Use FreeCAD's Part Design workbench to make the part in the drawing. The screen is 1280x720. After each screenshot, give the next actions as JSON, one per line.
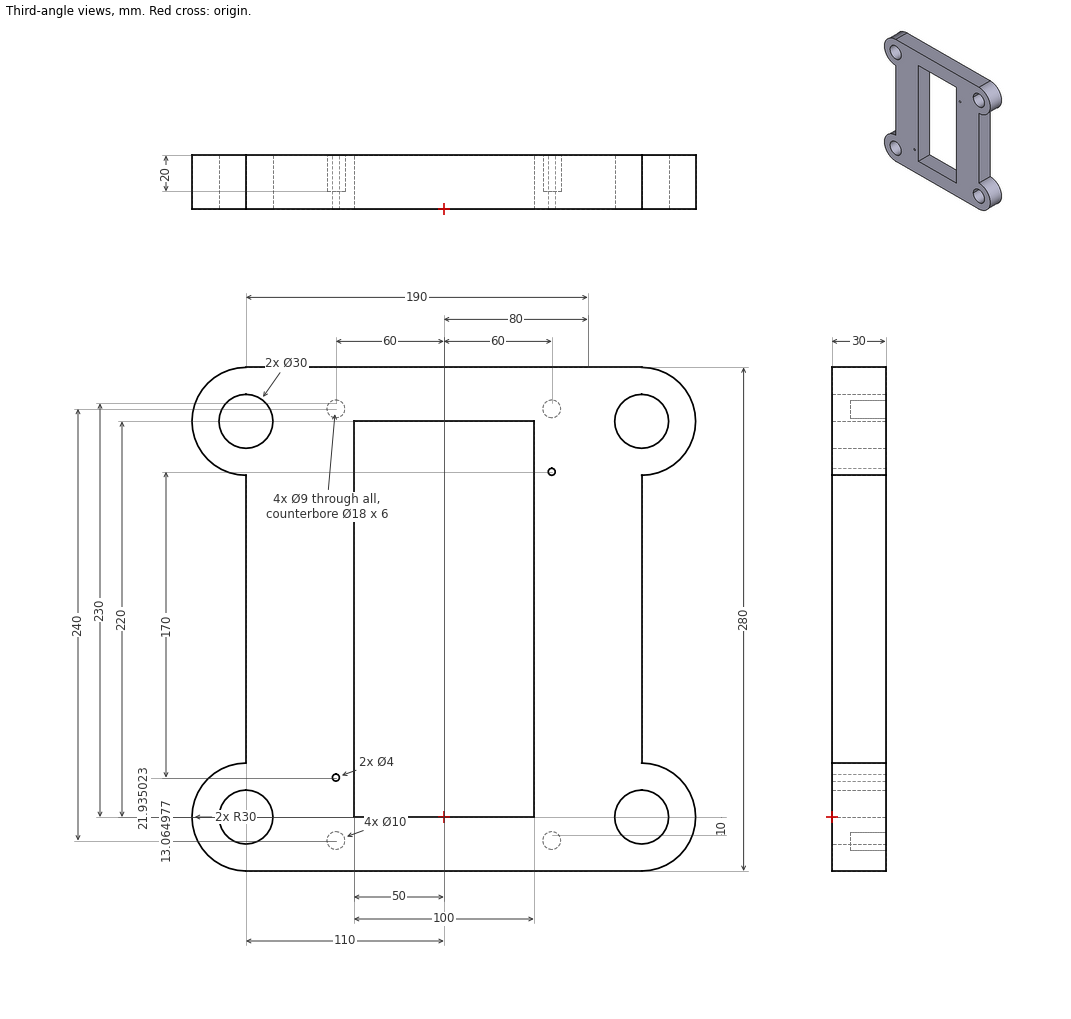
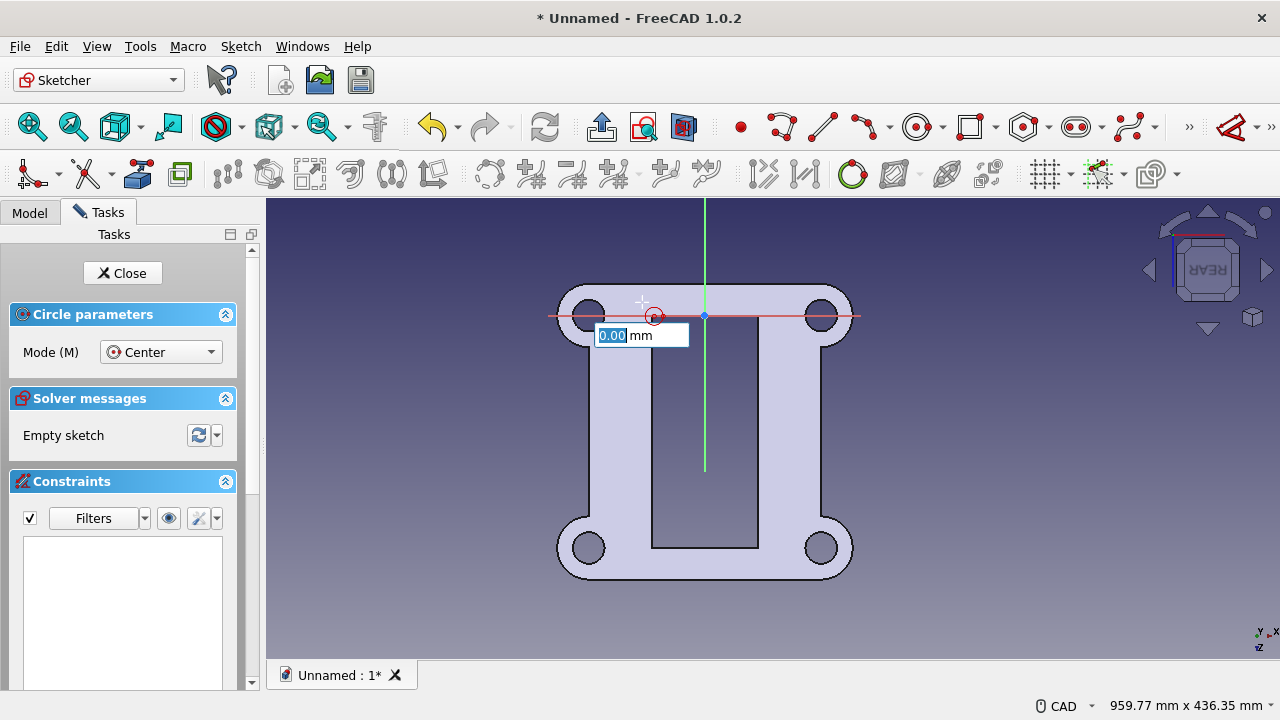
{"action": "scroll", "coordinate": [645, 298], "scroll_direction": "up", "scroll_amount": 6}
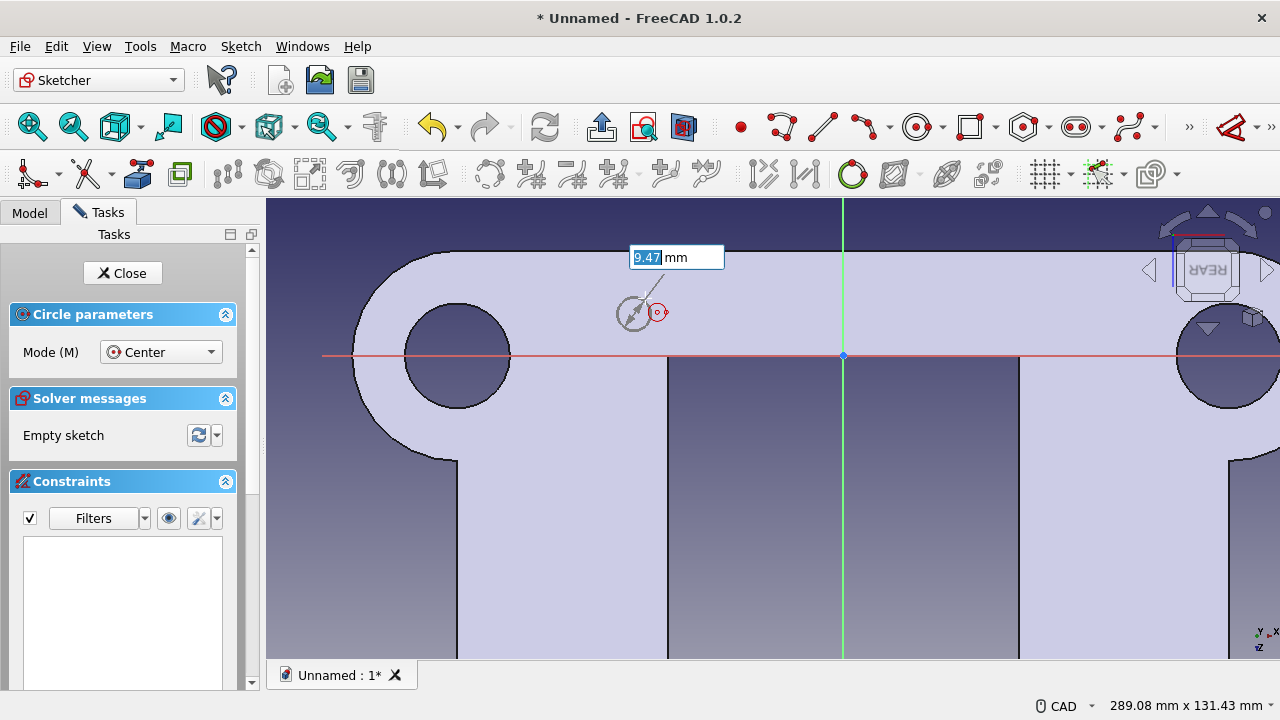
{"action": "left_click", "coordinate": [645, 298]}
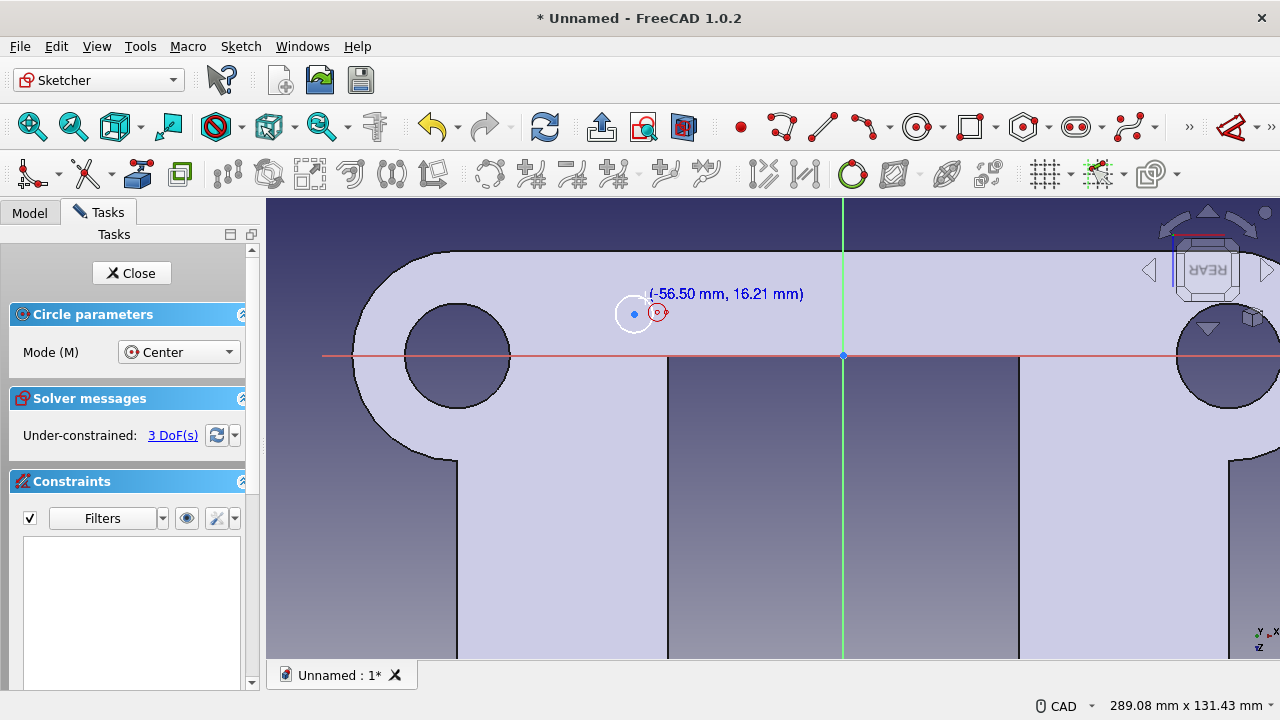
{"action": "scroll", "coordinate": [645, 298], "scroll_direction": "down", "scroll_amount": 6}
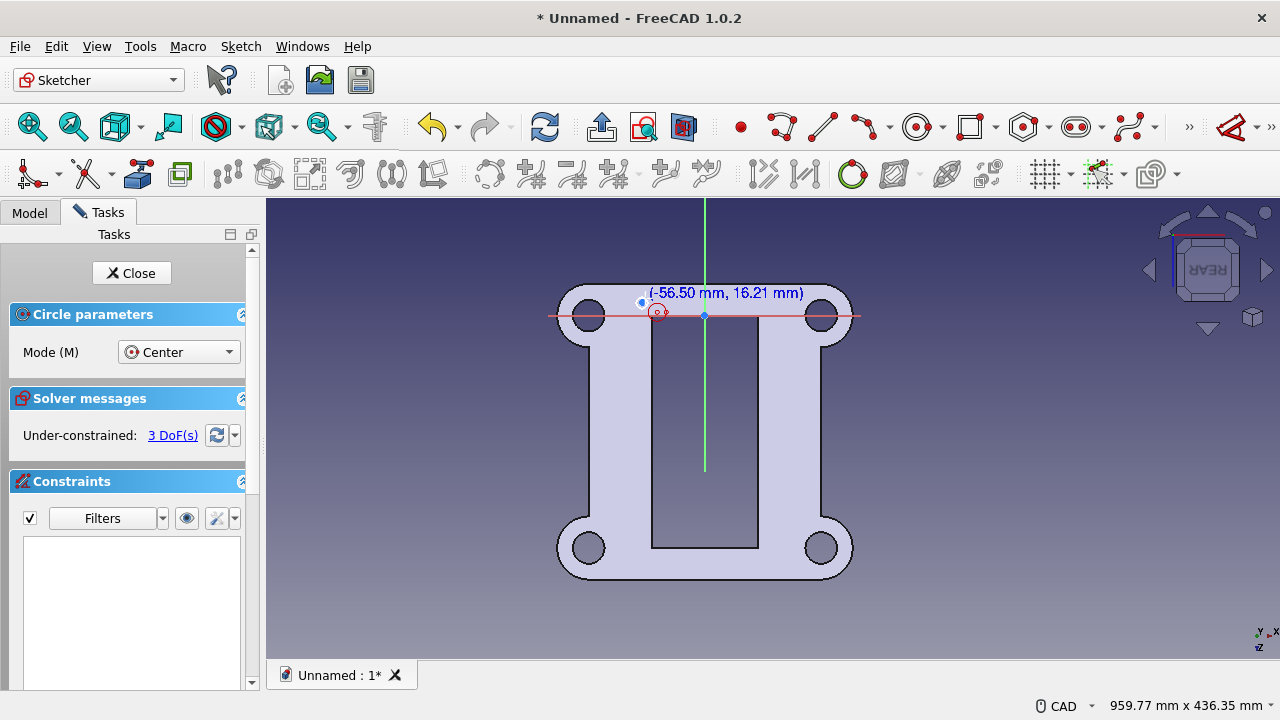
{"action": "scroll", "coordinate": [642, 555], "scroll_direction": "up", "scroll_amount": 8}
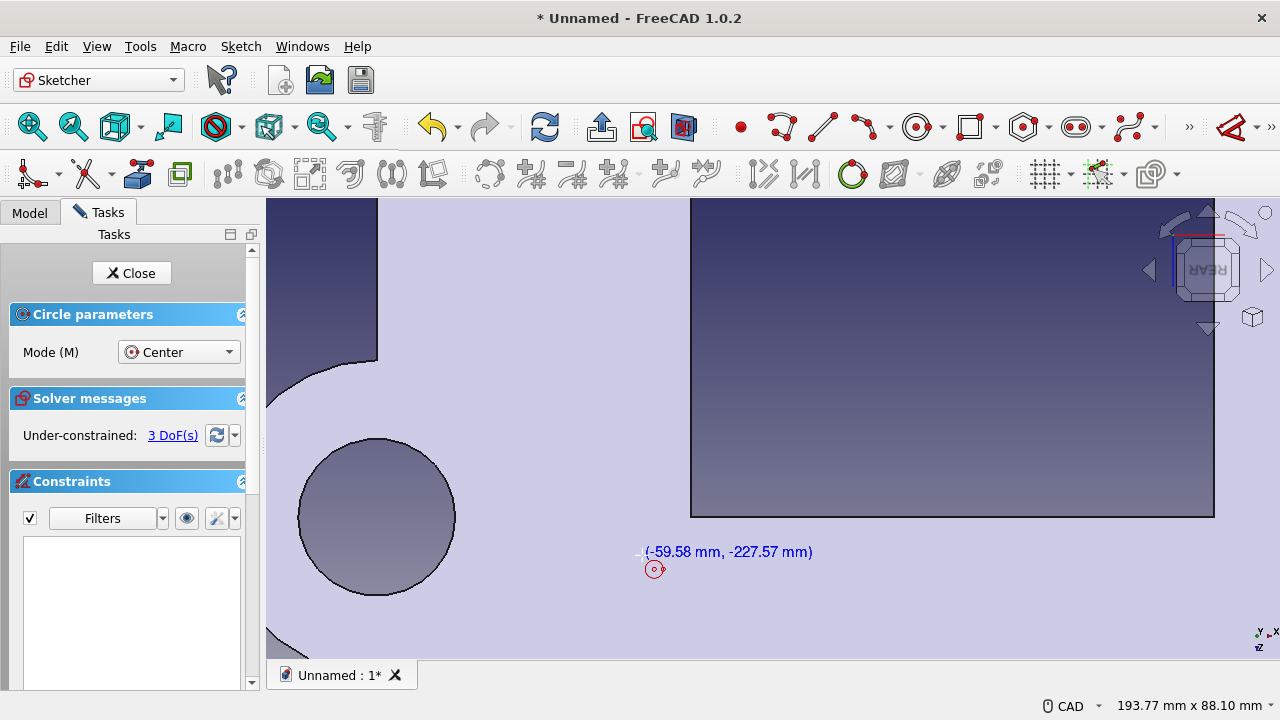
{"action": "scroll", "coordinate": [642, 556], "scroll_direction": "down", "scroll_amount": 8}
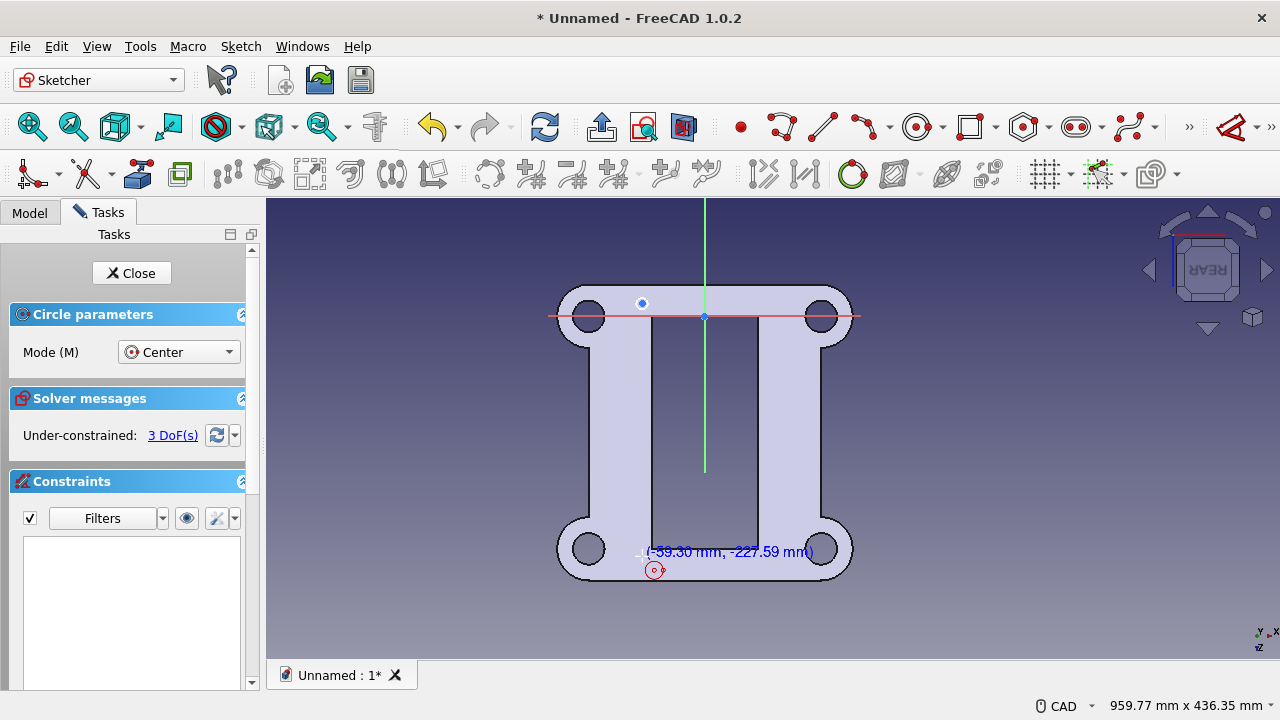
{"action": "left_click", "coordinate": [642, 556]}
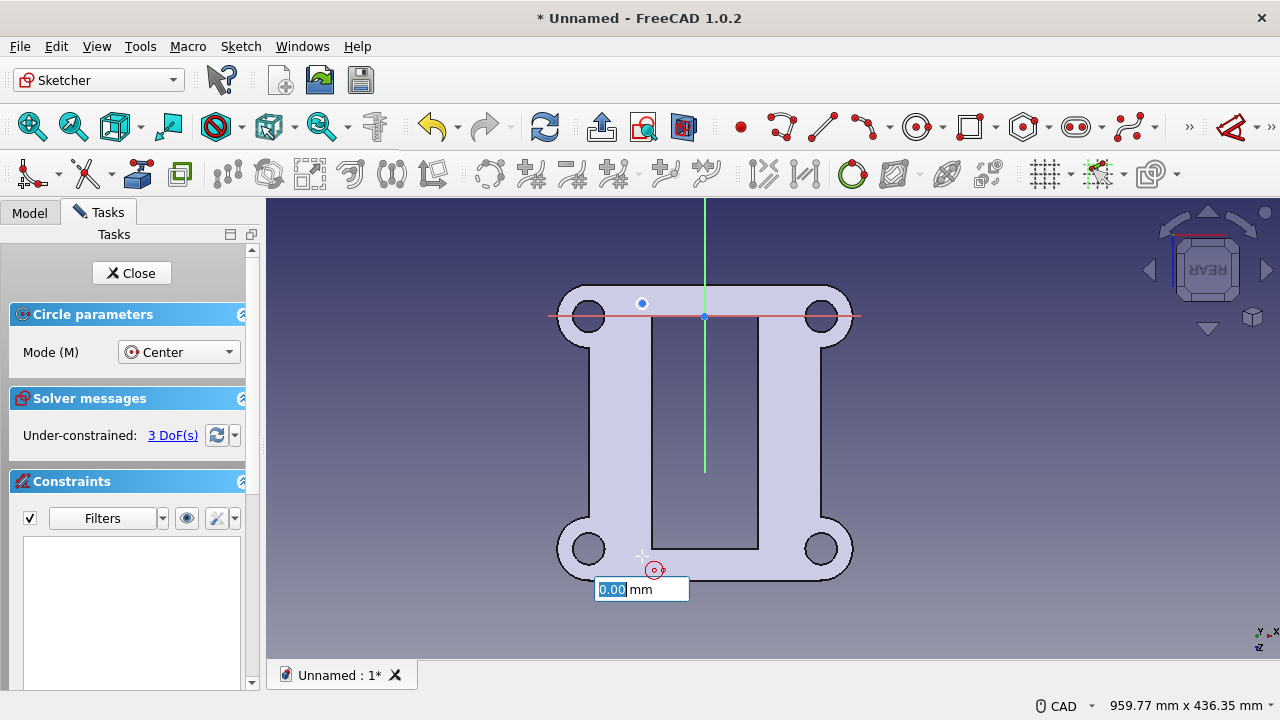
{"action": "scroll", "coordinate": [645, 552], "scroll_direction": "up", "scroll_amount": 6}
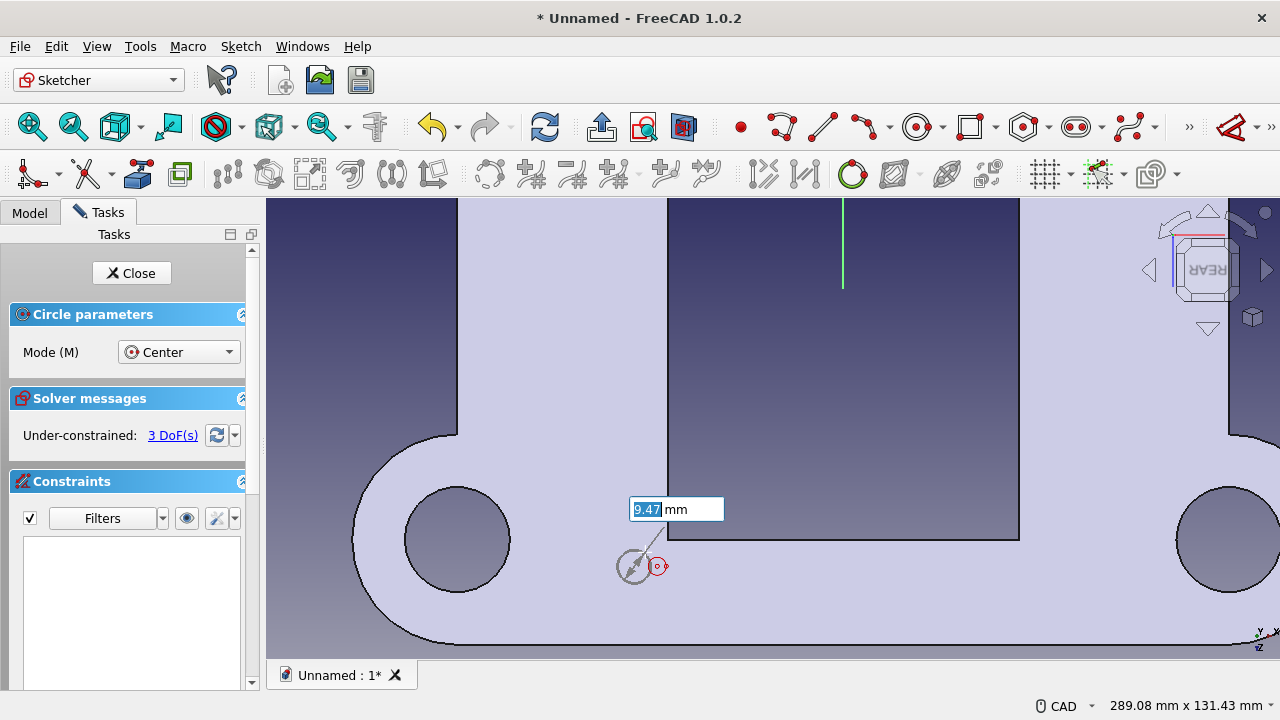
{"action": "left_click", "coordinate": [645, 552]}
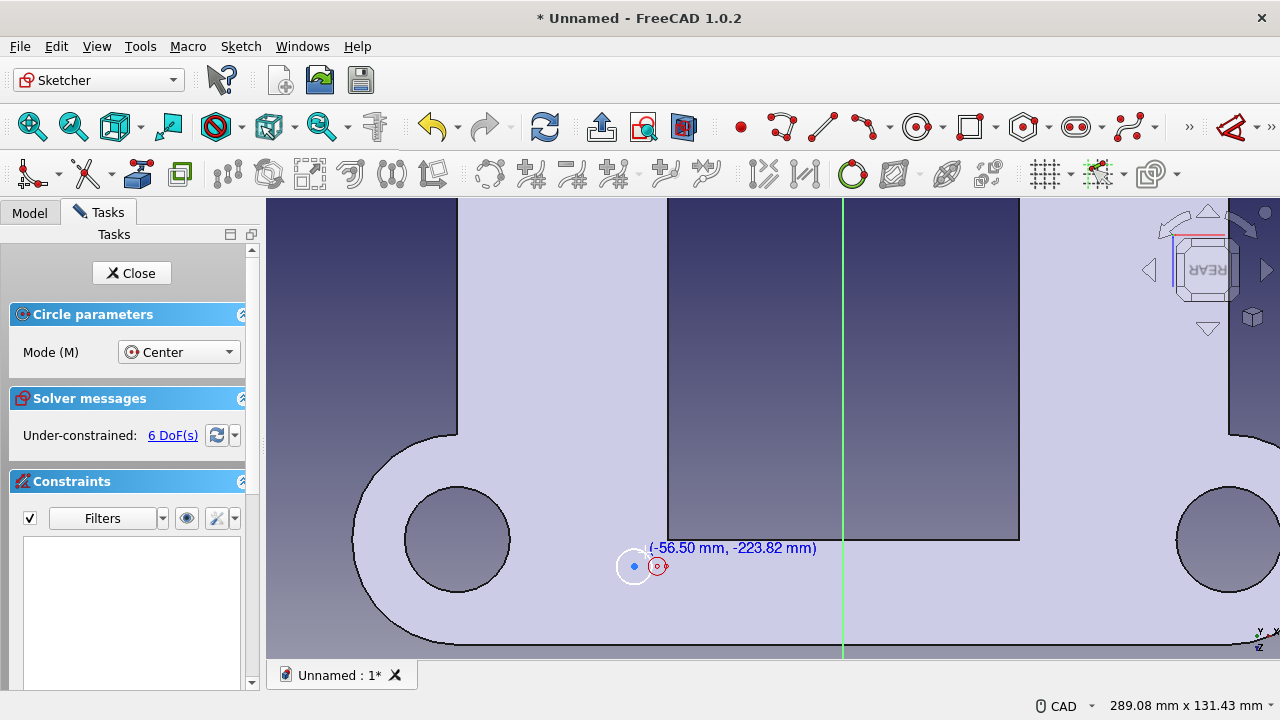
{"action": "scroll", "coordinate": [645, 552], "scroll_direction": "down", "scroll_amount": 6}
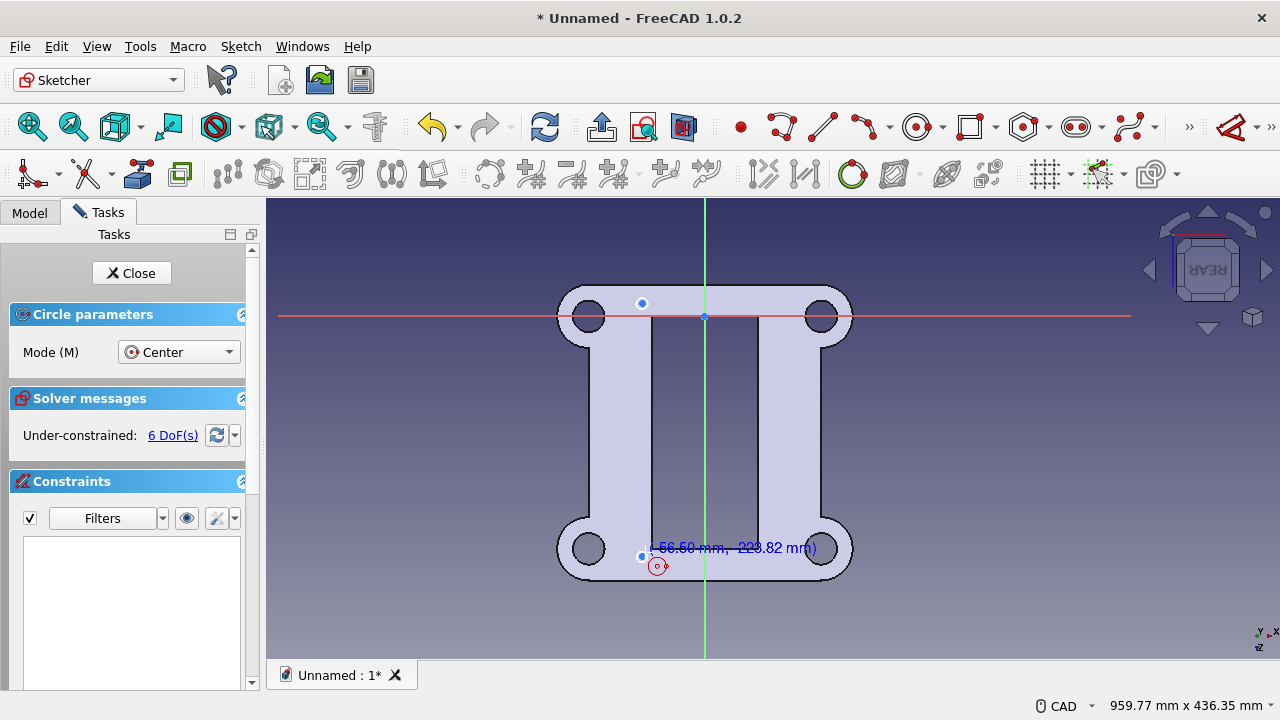
{"action": "scroll", "coordinate": [768, 303], "scroll_direction": "up", "scroll_amount": 8}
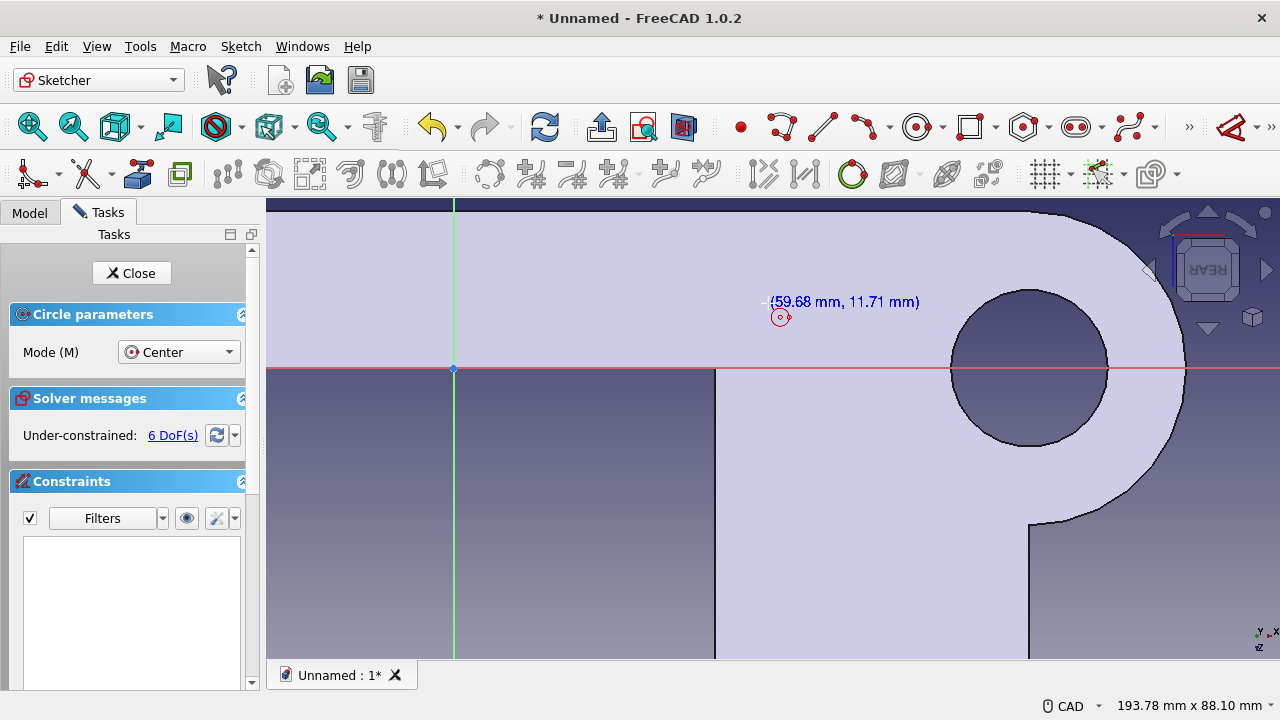
{"action": "scroll", "coordinate": [768, 302], "scroll_direction": "down", "scroll_amount": 8}